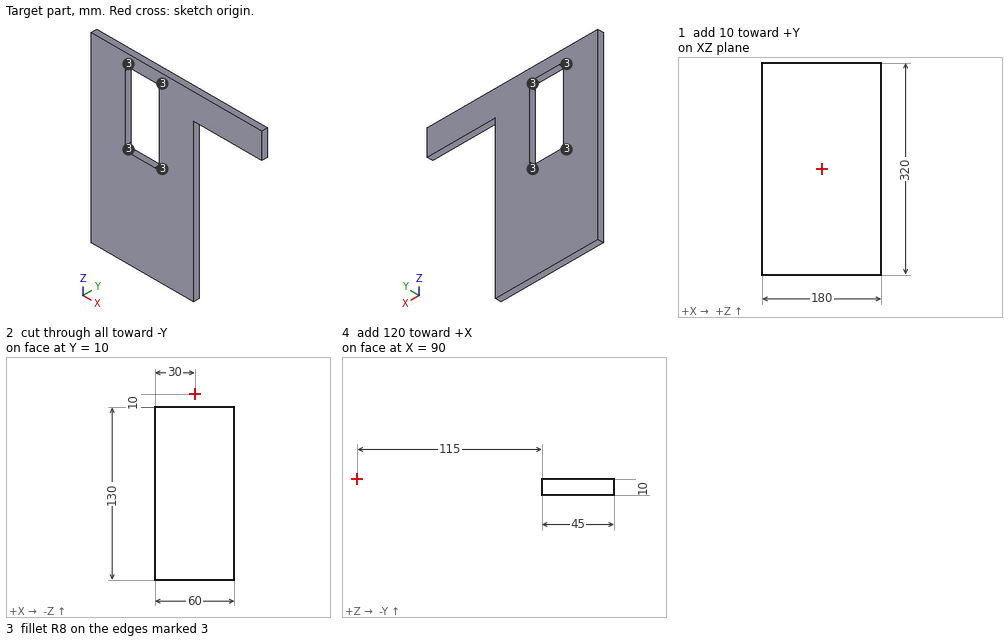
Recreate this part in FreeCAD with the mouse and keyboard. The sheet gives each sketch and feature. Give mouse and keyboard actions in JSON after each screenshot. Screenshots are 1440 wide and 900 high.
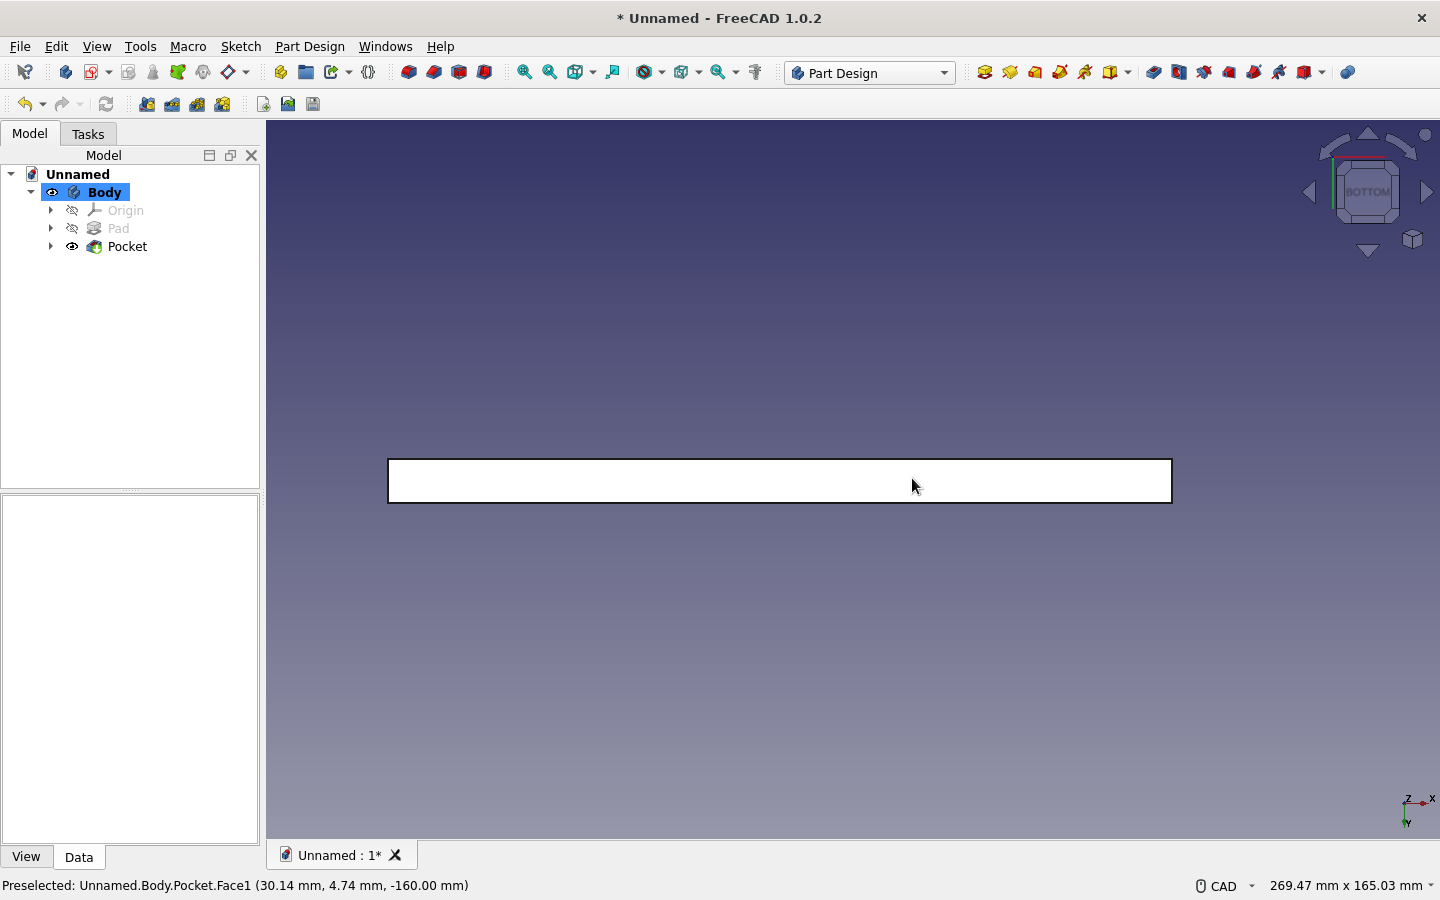
{"action": "key", "text": "v f"}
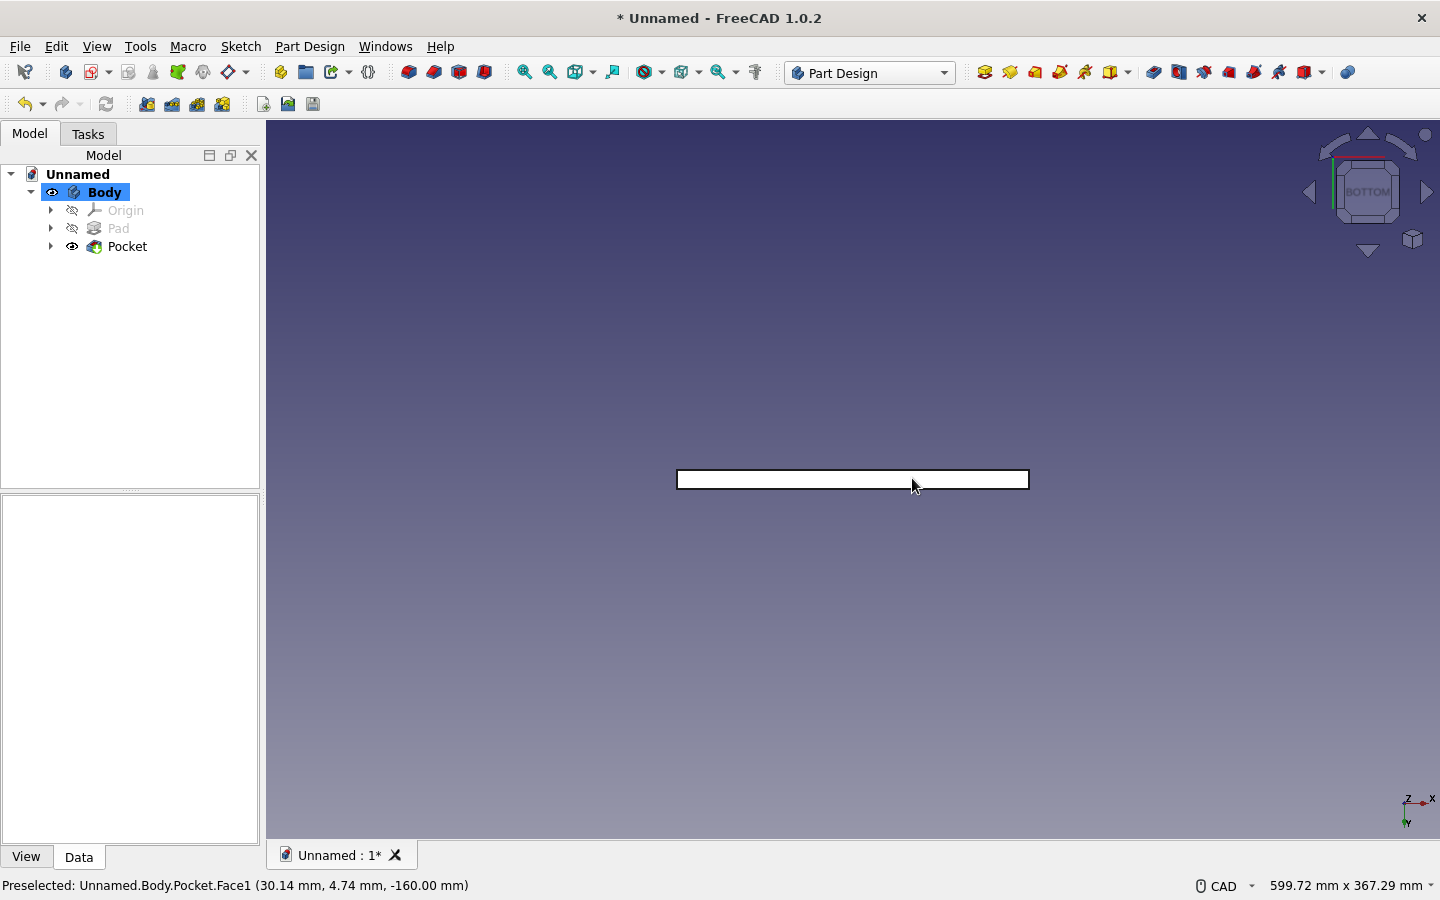
{"action": "key", "text": "4"}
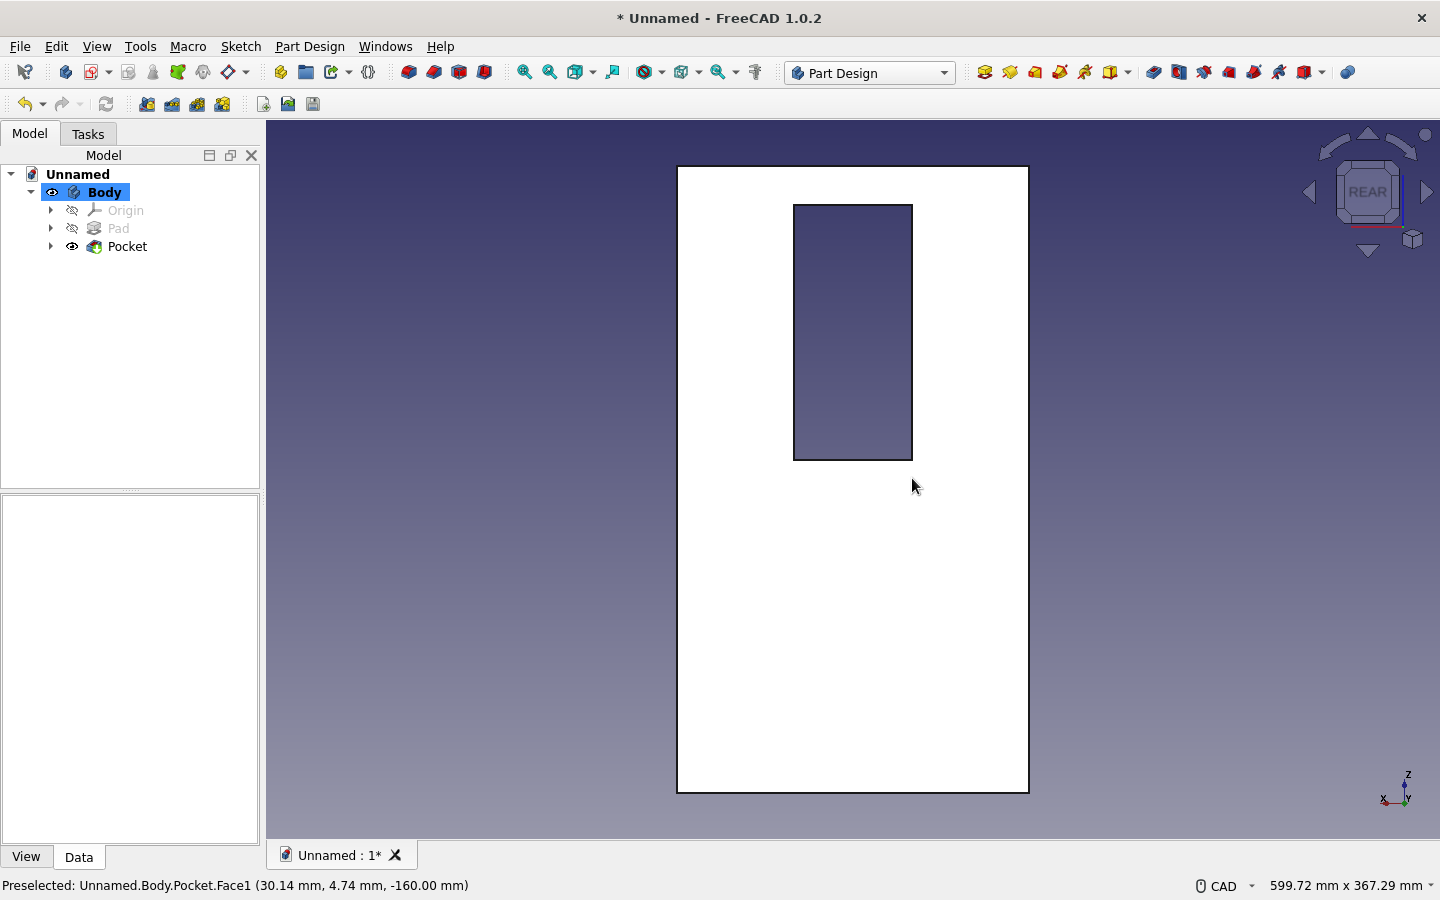
{"action": "scroll", "coordinate": [794, 459], "scroll_direction": "up", "scroll_amount": 4}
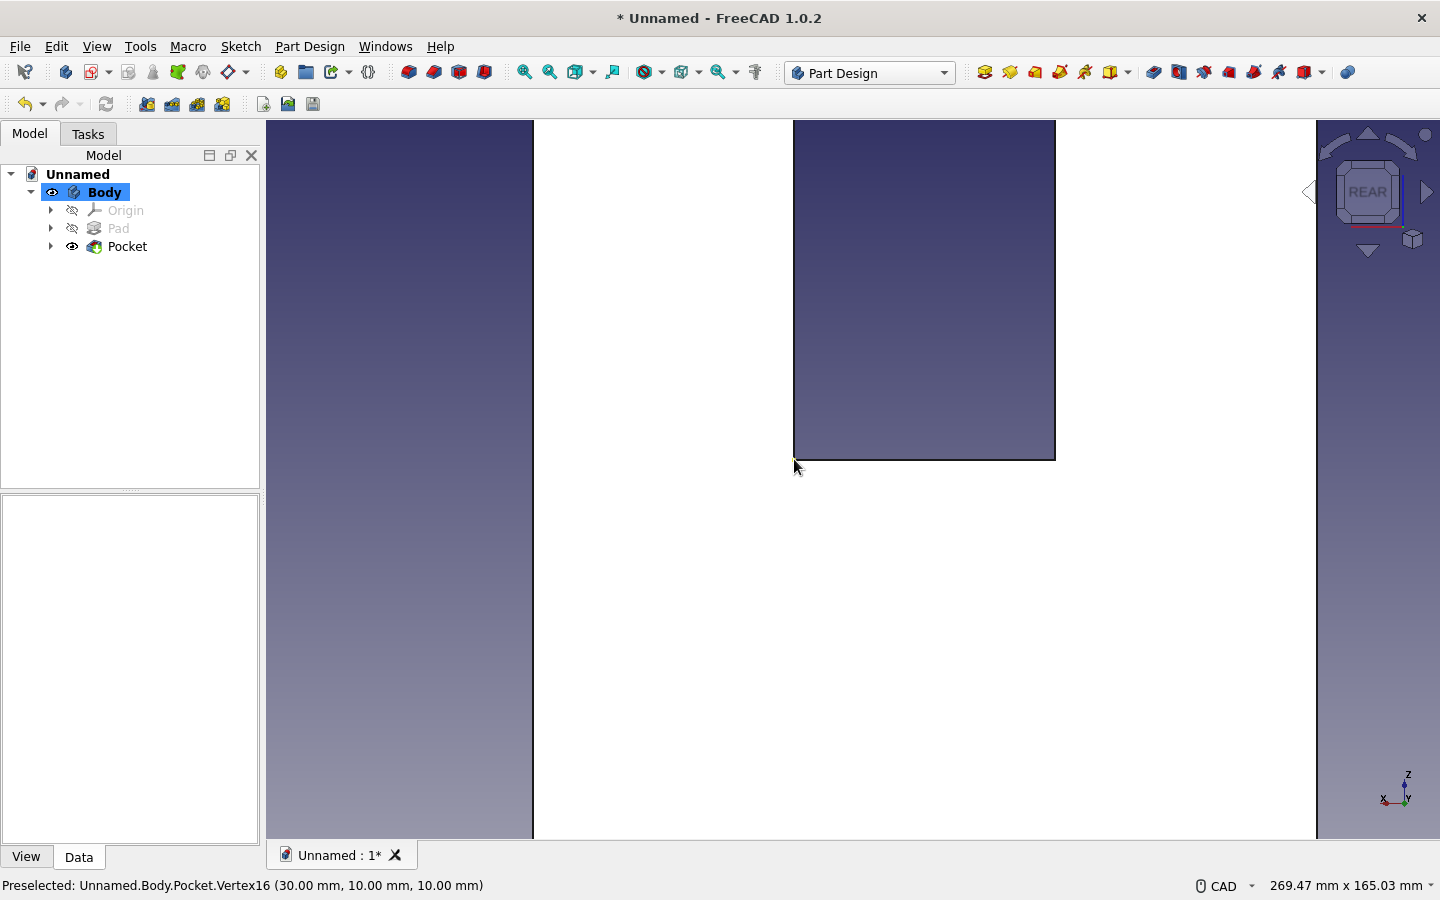
{"action": "key", "text": "v f"}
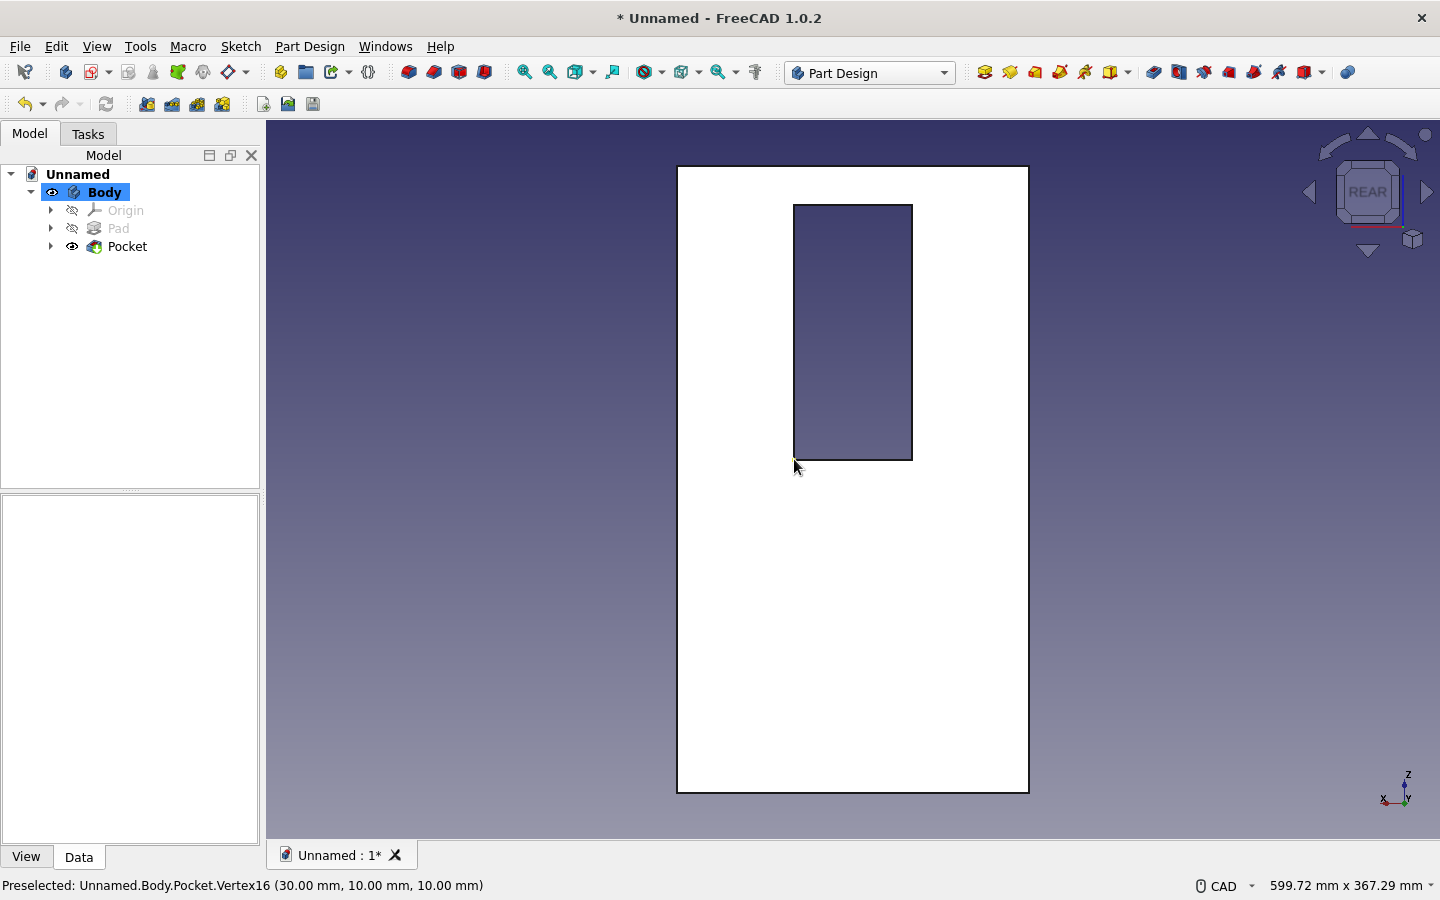
{"action": "key", "text": "6"}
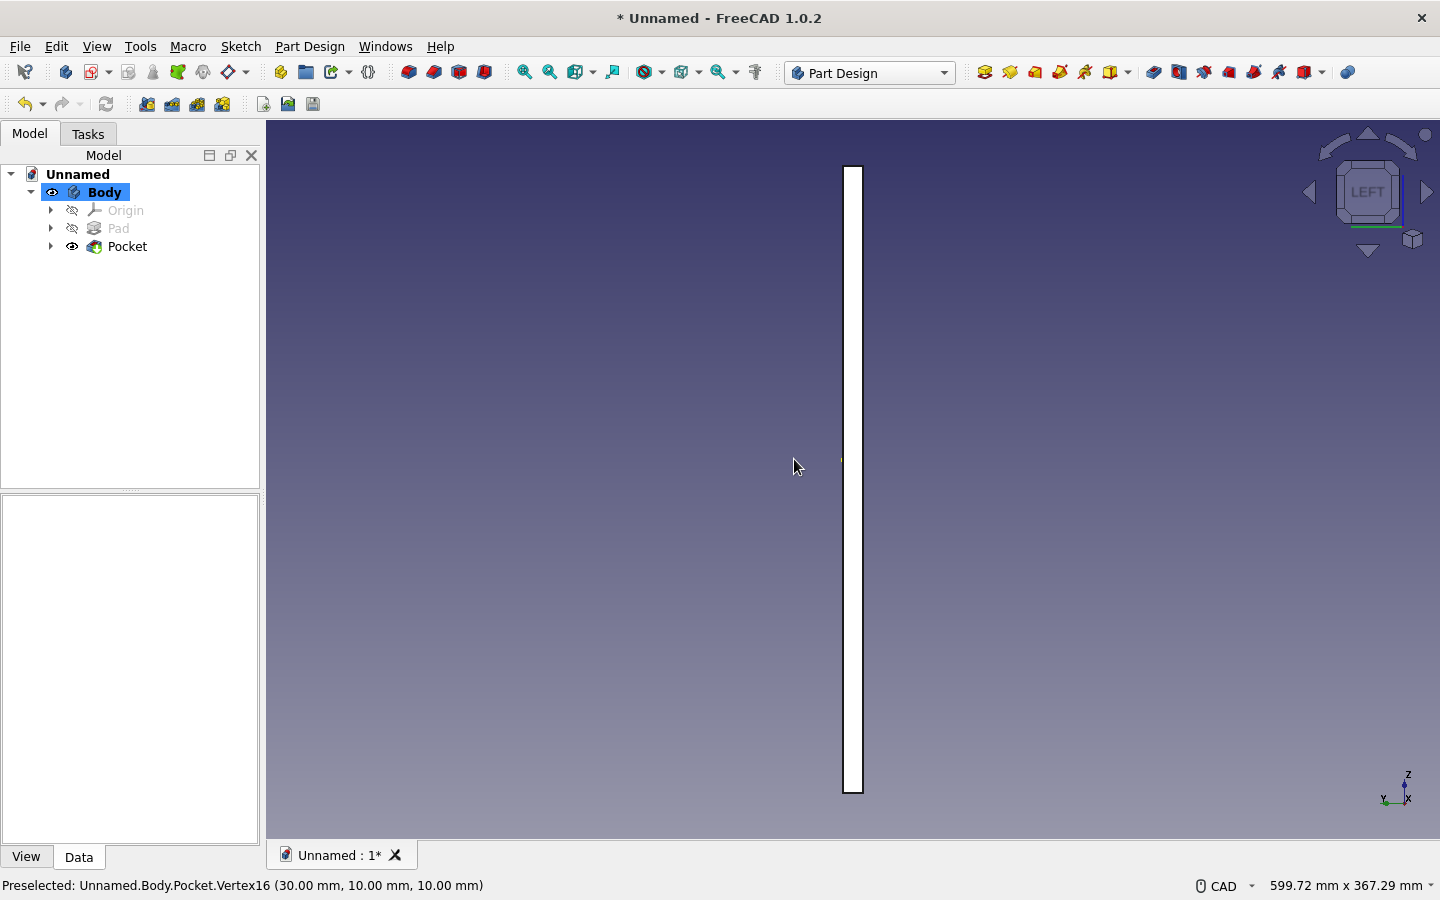
{"action": "scroll", "coordinate": [853, 459], "scroll_direction": "up", "scroll_amount": 4}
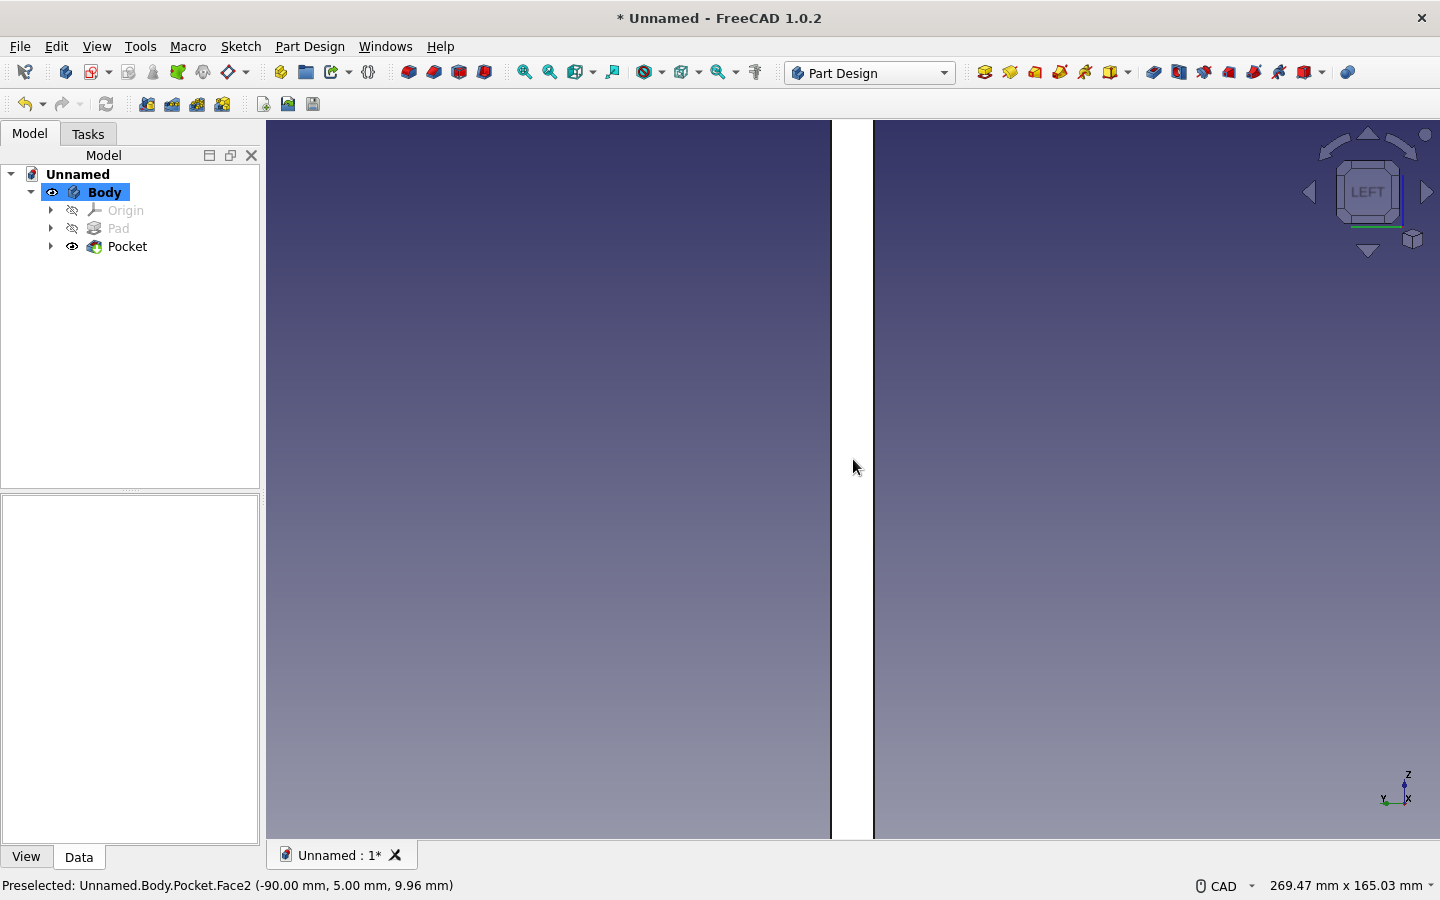
{"action": "key", "text": "v f"}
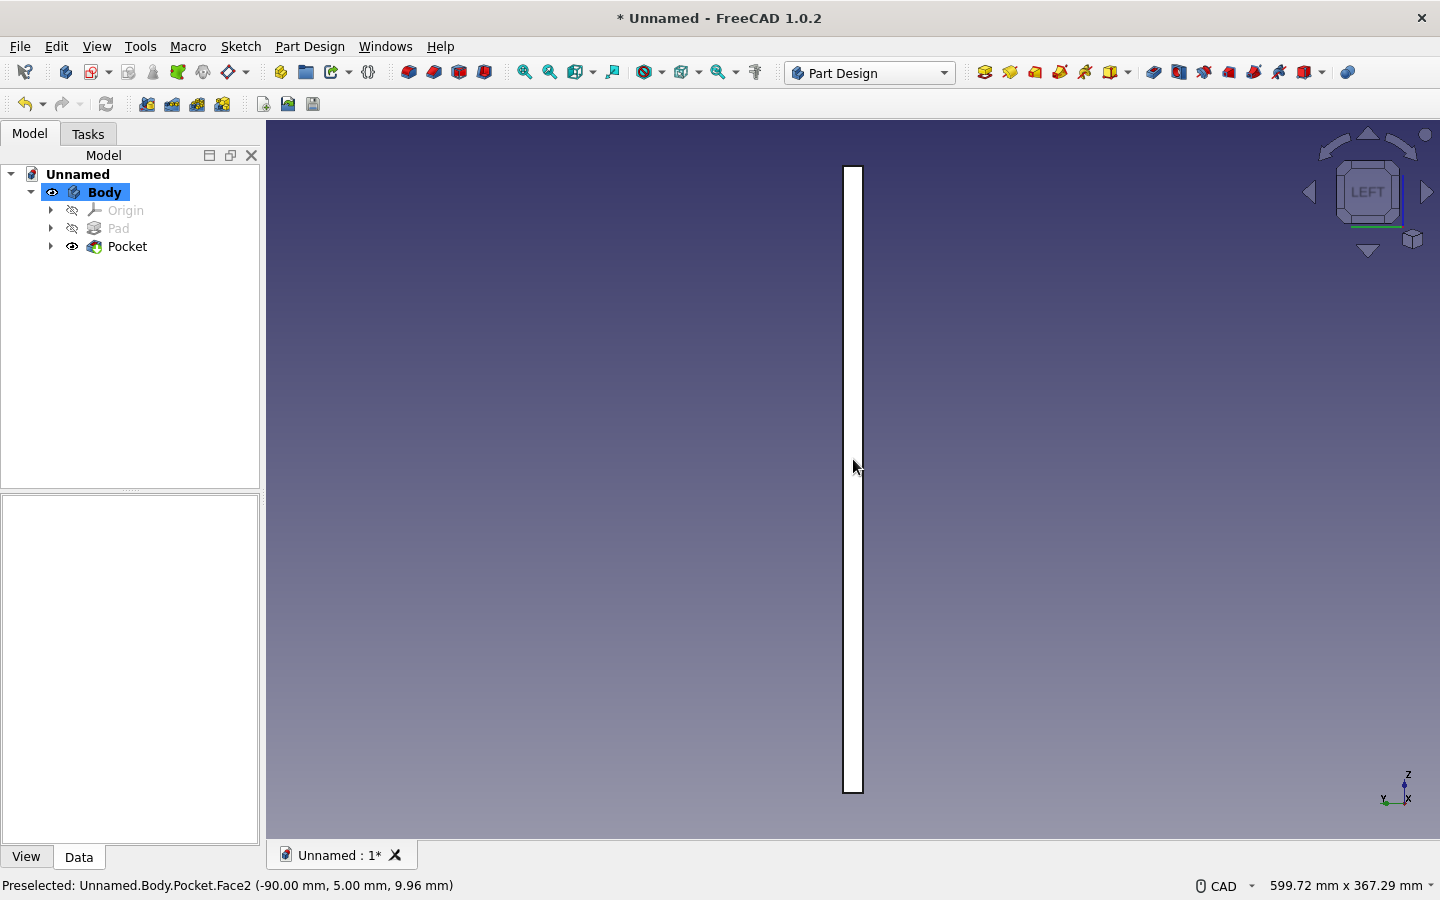
{"action": "key", "text": "v 3"}